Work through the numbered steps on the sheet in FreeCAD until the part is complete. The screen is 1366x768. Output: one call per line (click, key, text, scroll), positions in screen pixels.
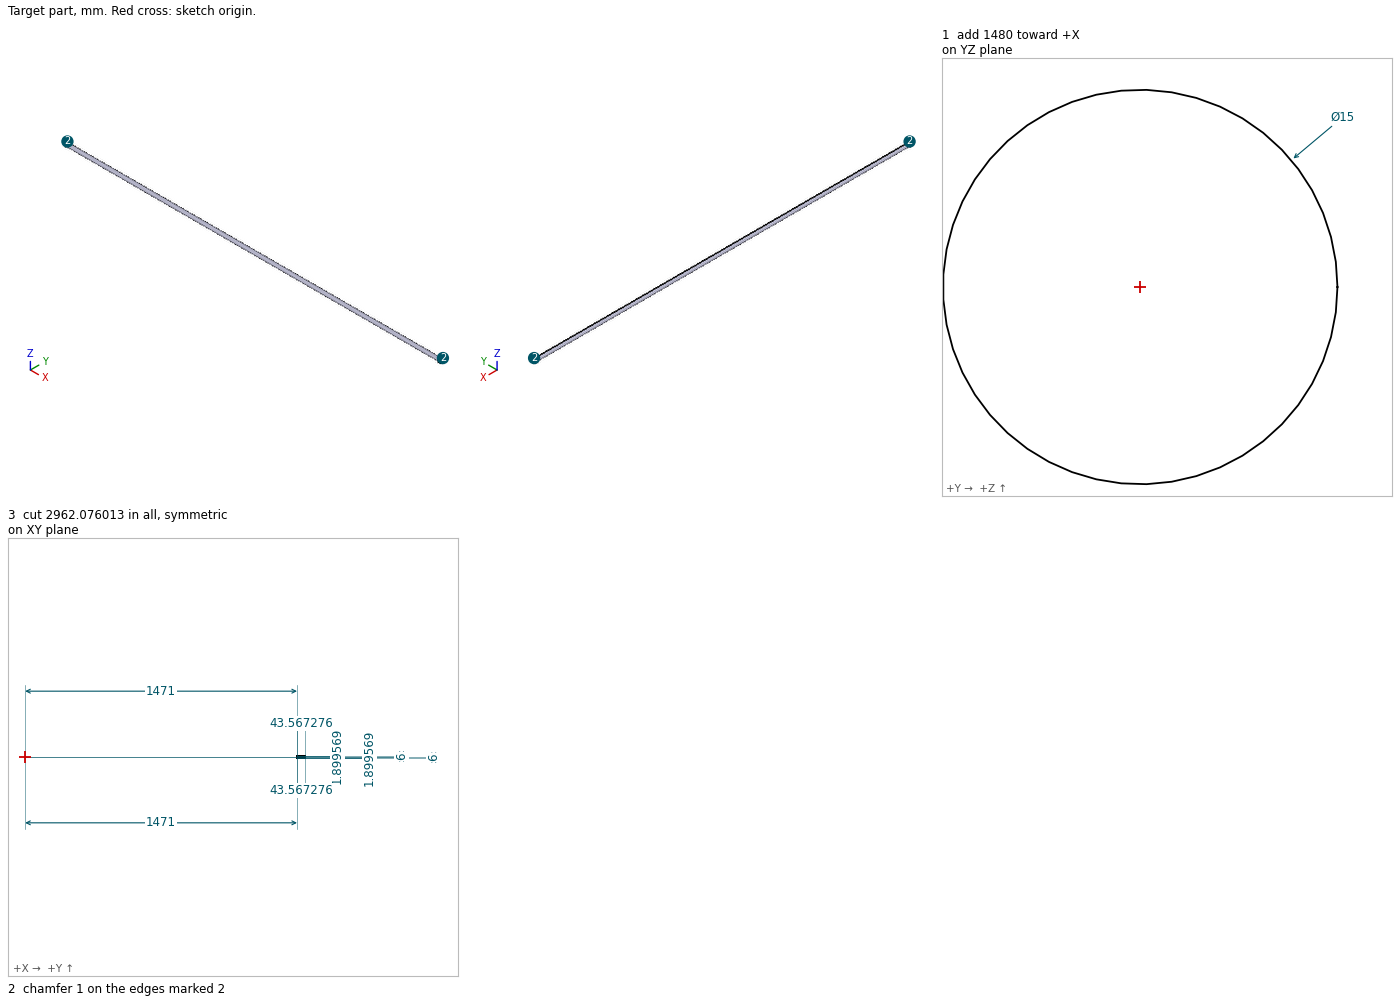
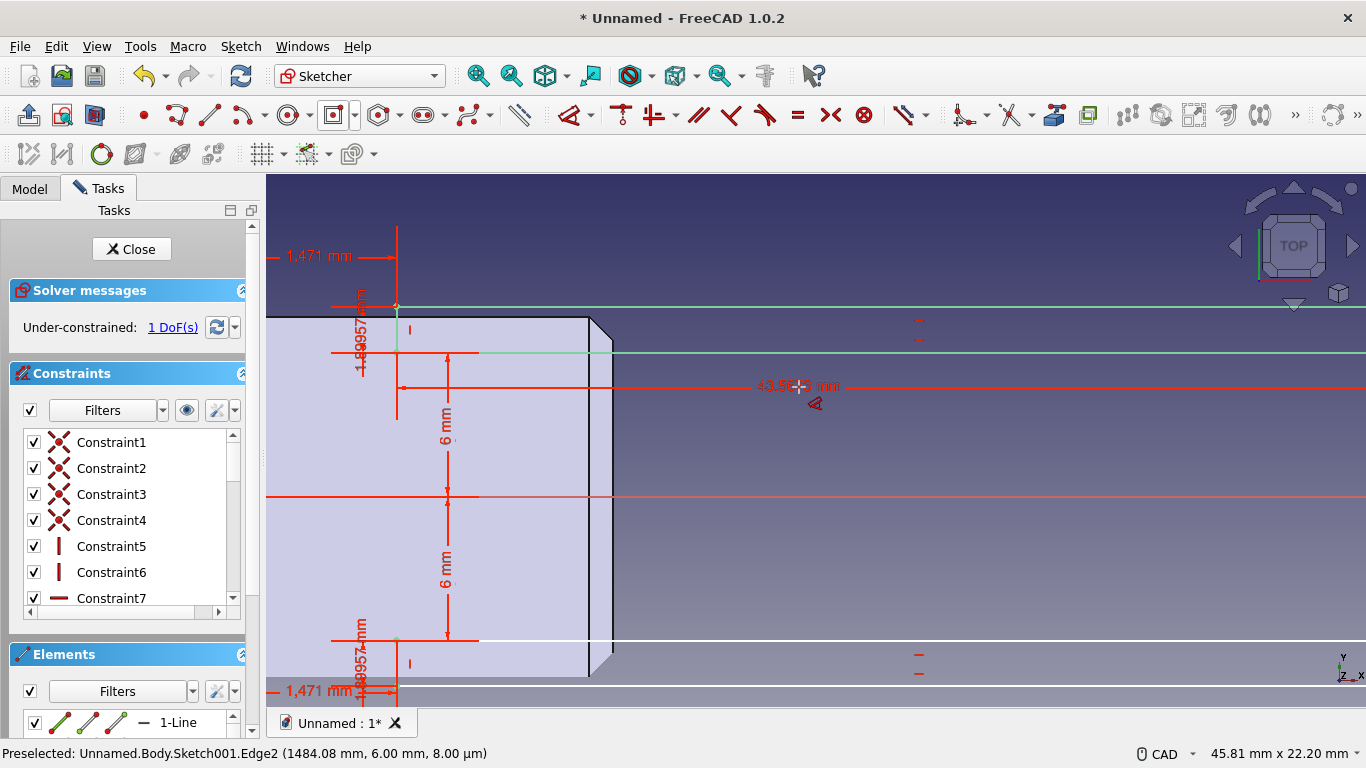
scroll(397, 326, down, 2)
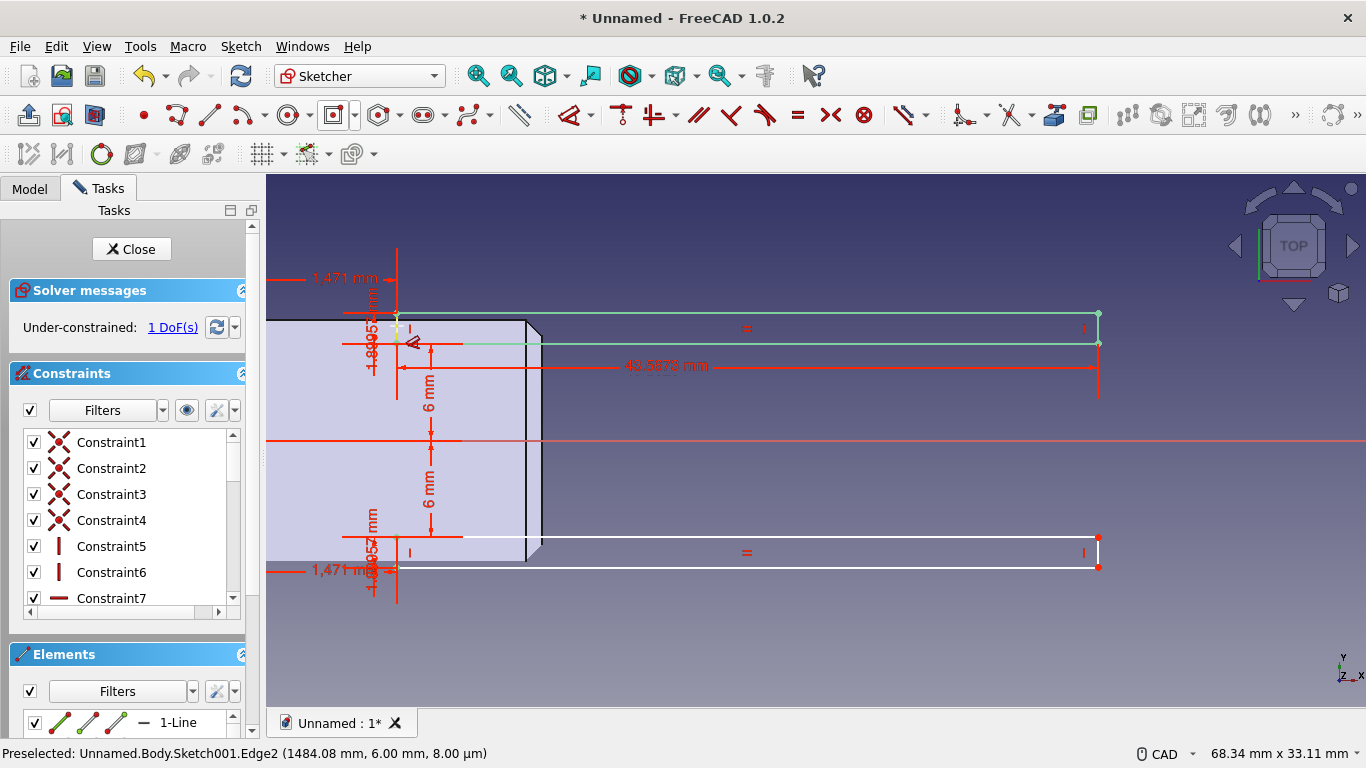
click(607, 568)
click(747, 602)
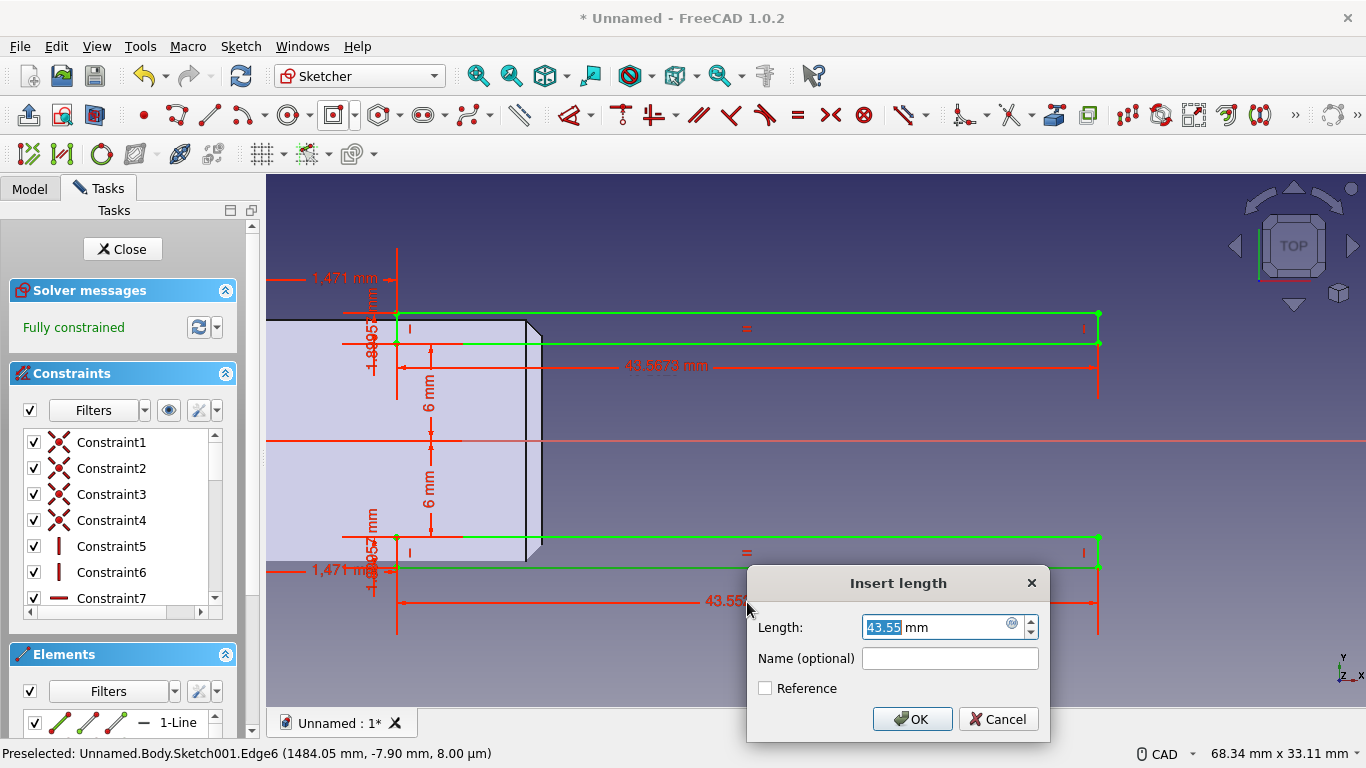
text(43.567276)
key(Return)
key(Escape)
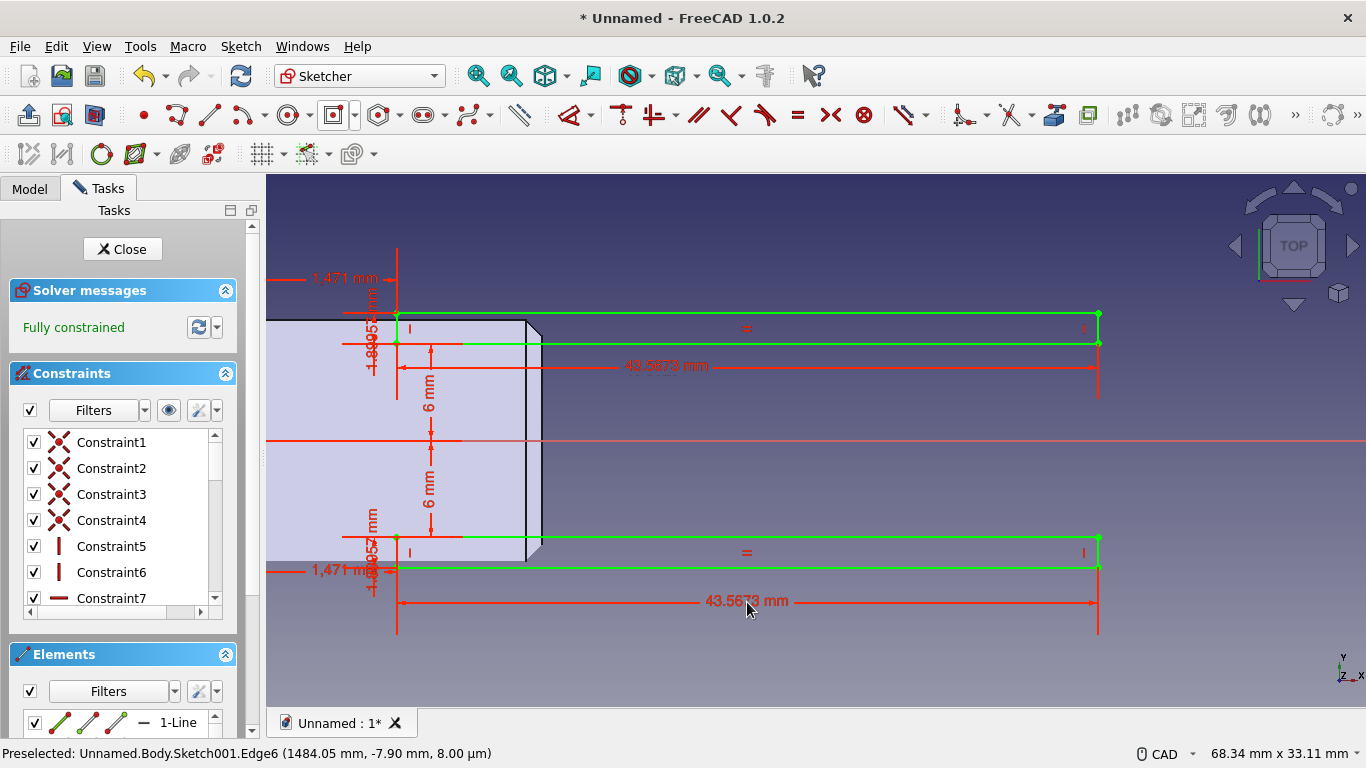
click(123, 249)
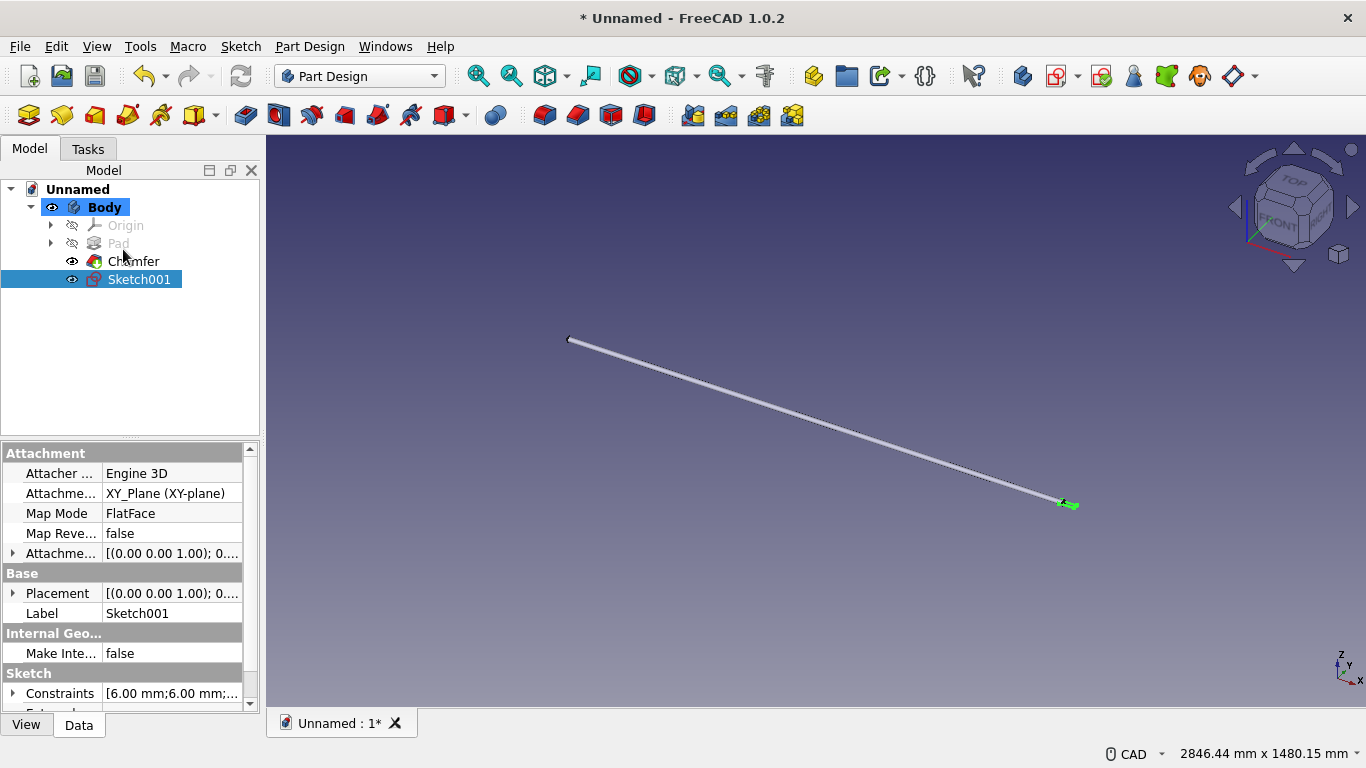
click(246, 116)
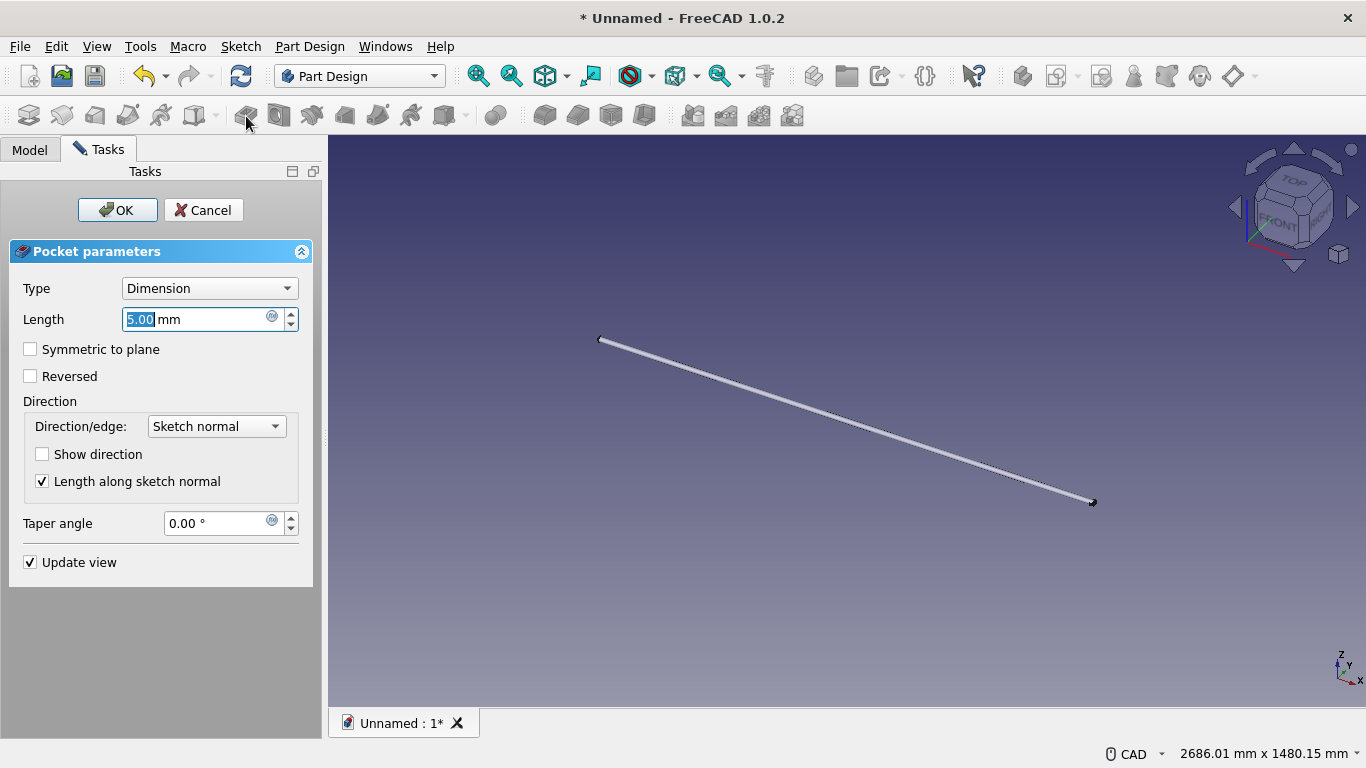
text(2962.076013)
key(Tab)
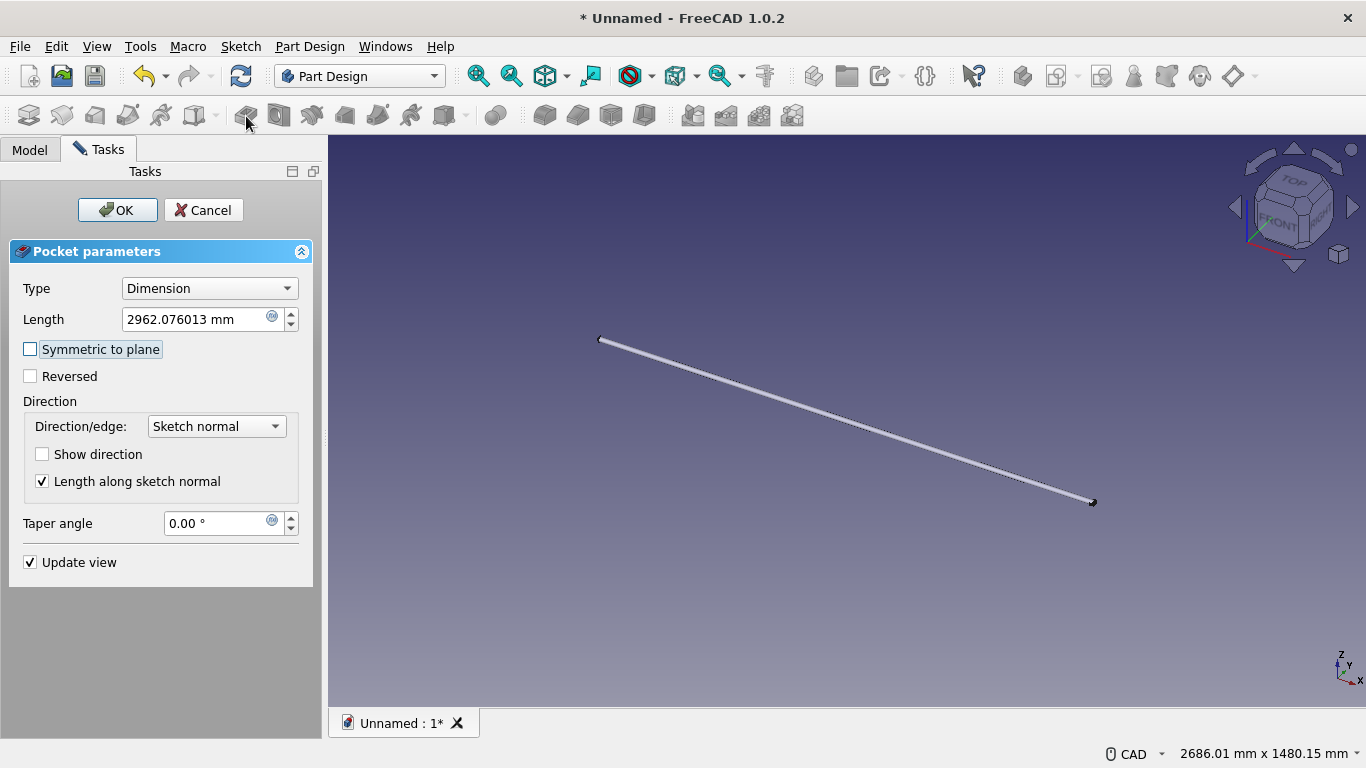
click(31, 349)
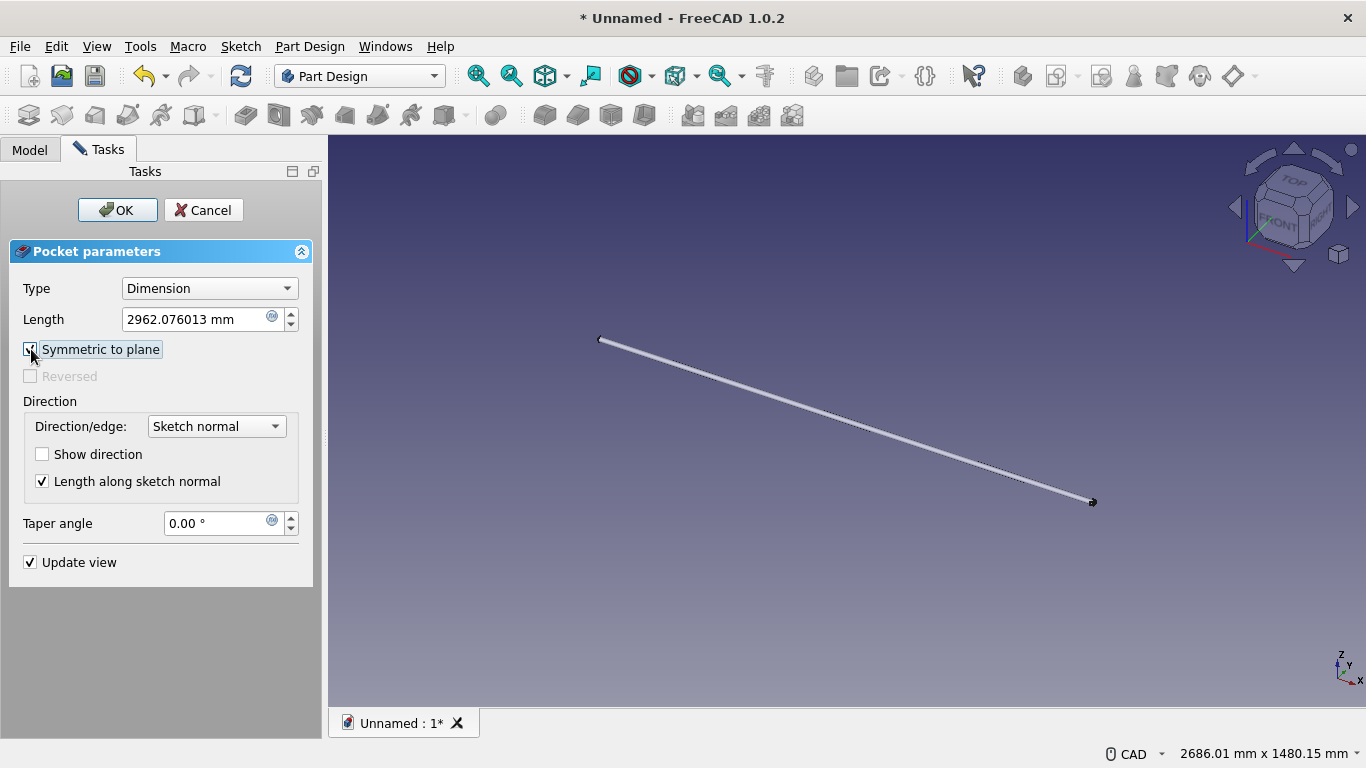
click(118, 210)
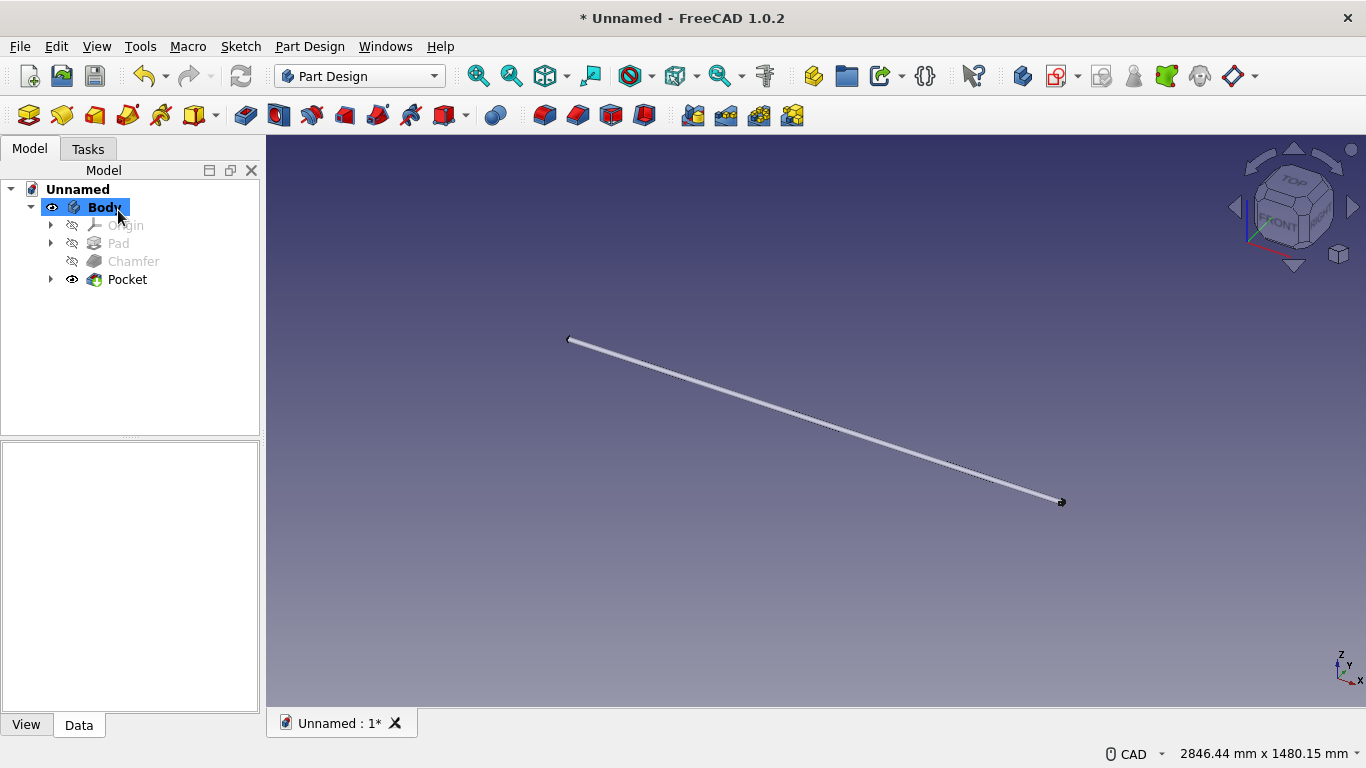
key(0)